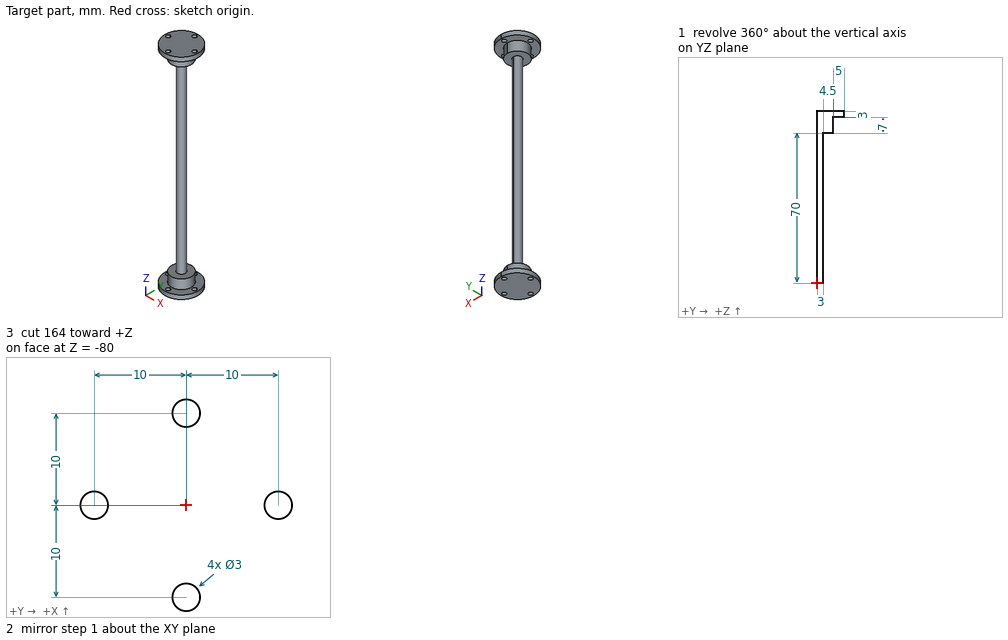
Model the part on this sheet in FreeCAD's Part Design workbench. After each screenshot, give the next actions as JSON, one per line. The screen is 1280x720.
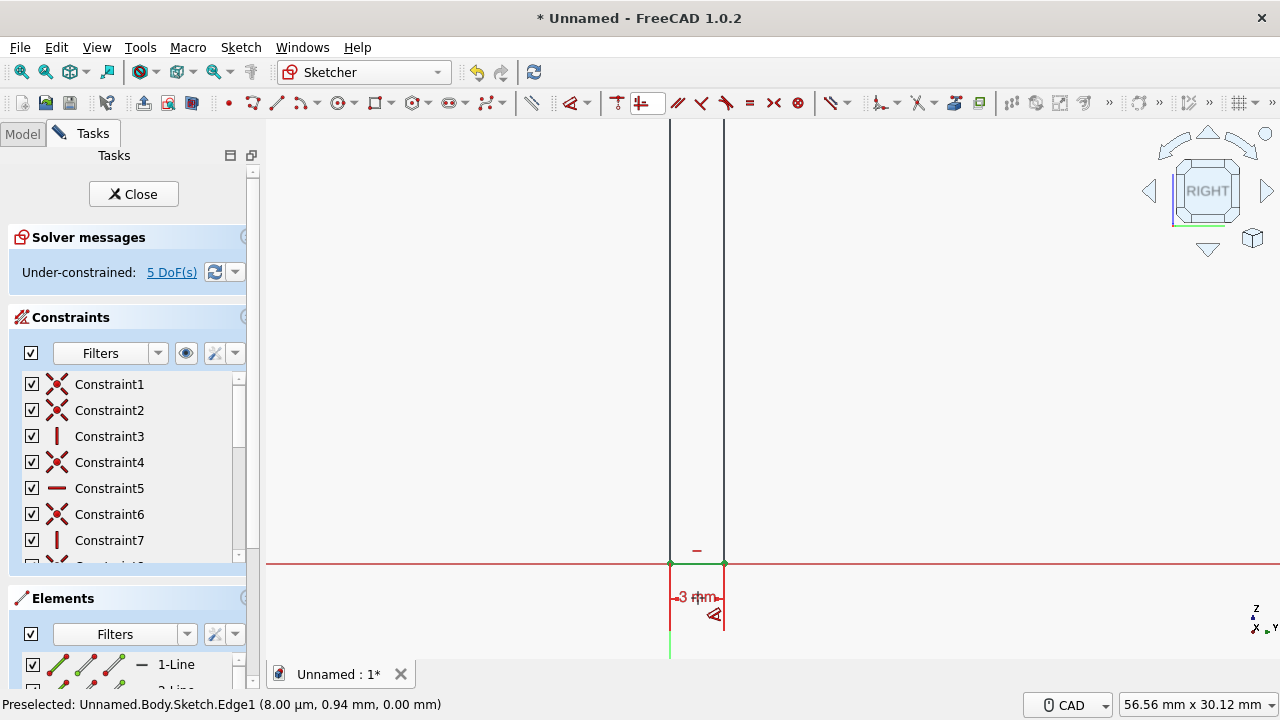
{"action": "scroll", "coordinate": [679, 567], "scroll_direction": "down", "scroll_amount": 7}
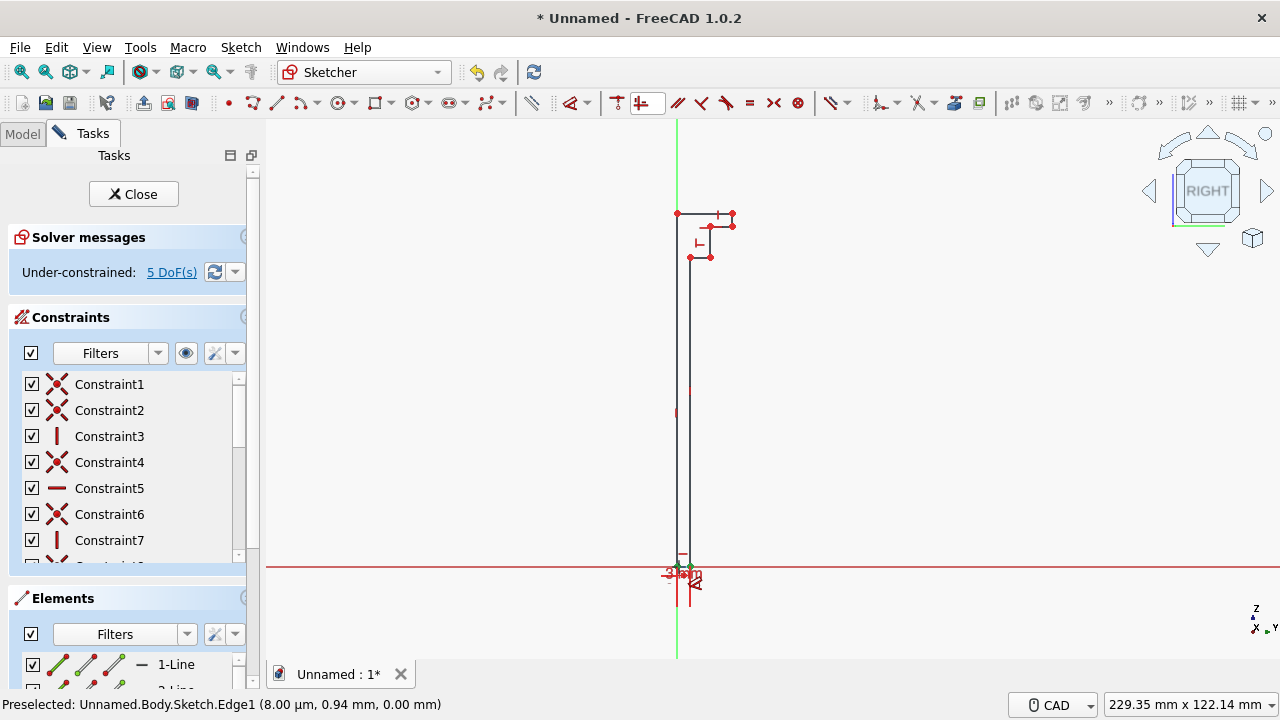
{"action": "scroll", "coordinate": [710, 249], "scroll_direction": "up", "scroll_amount": 2}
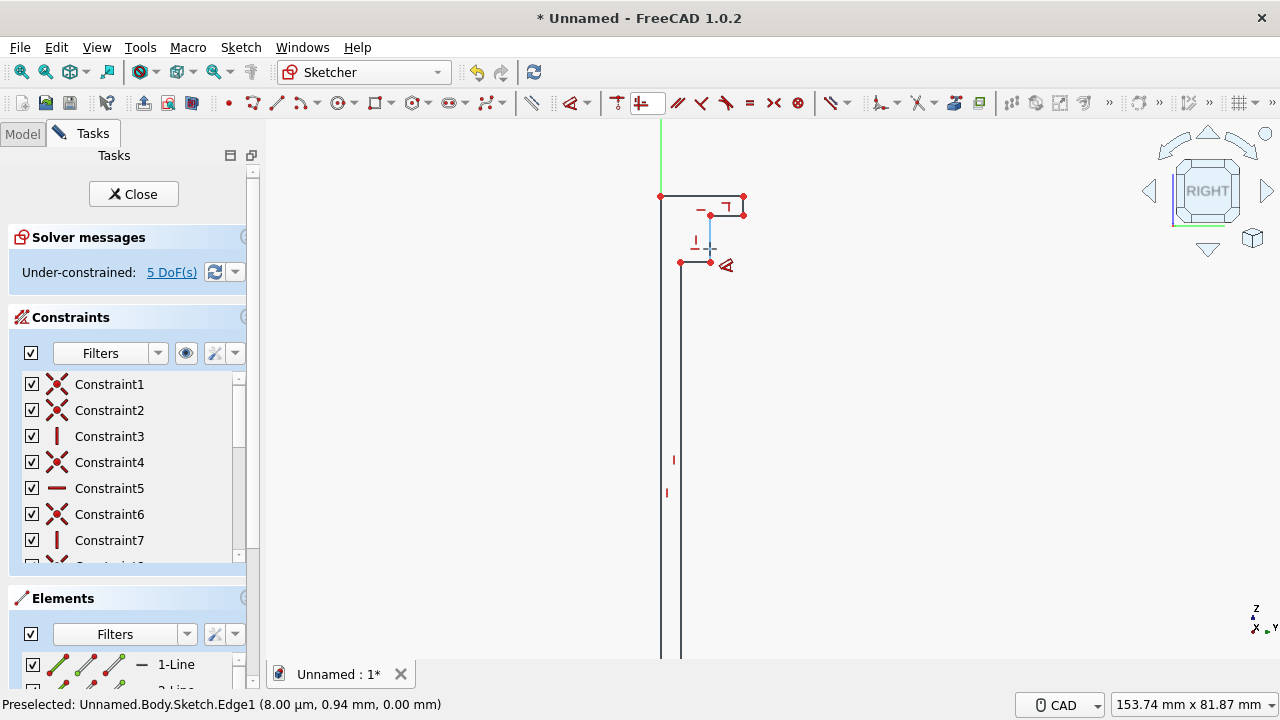
{"action": "left_click", "coordinate": [710, 248]}
{"action": "left_click", "coordinate": [744, 239]}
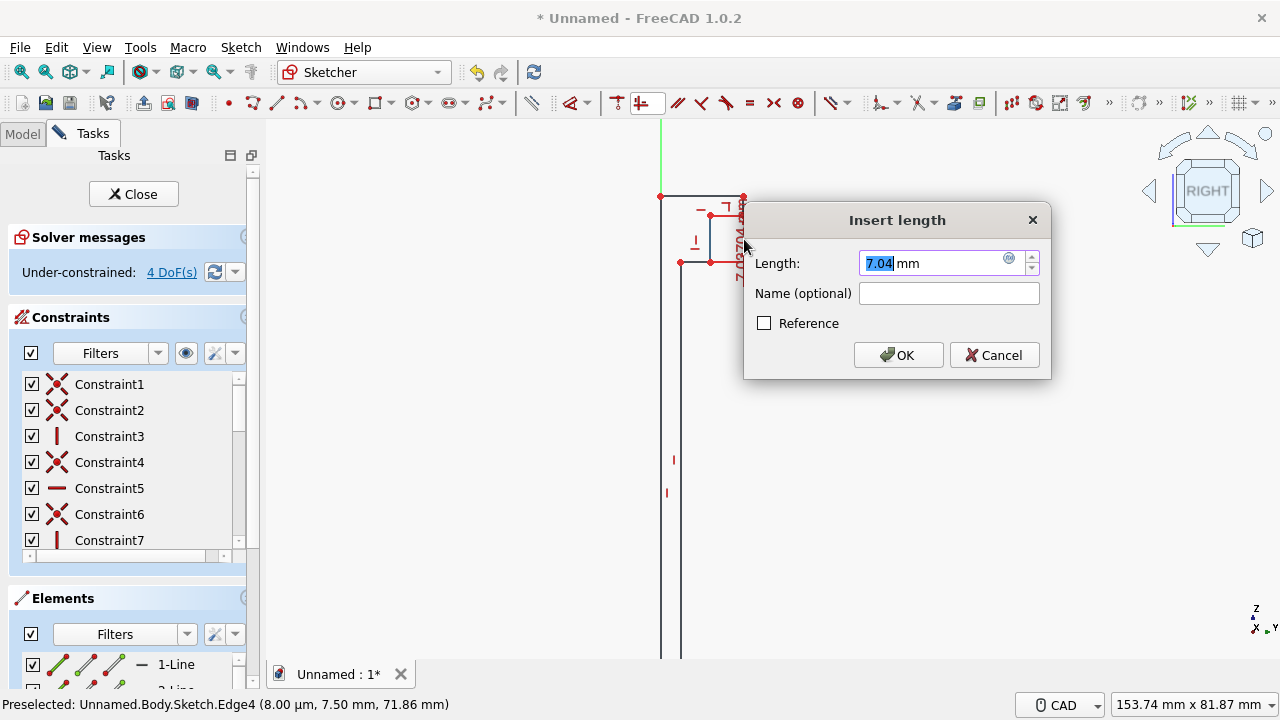
{"action": "type", "text": "7"}
{"action": "key", "text": "Return"}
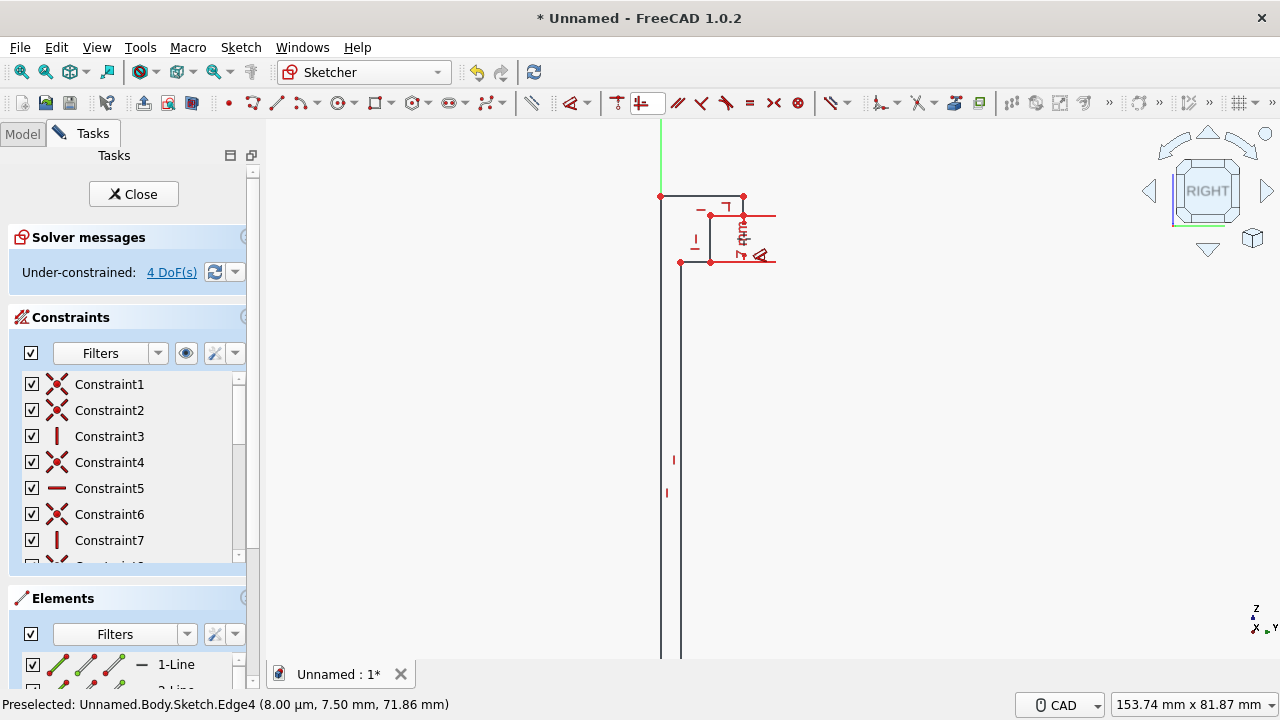
{"action": "scroll", "coordinate": [720, 216], "scroll_direction": "up", "scroll_amount": 2}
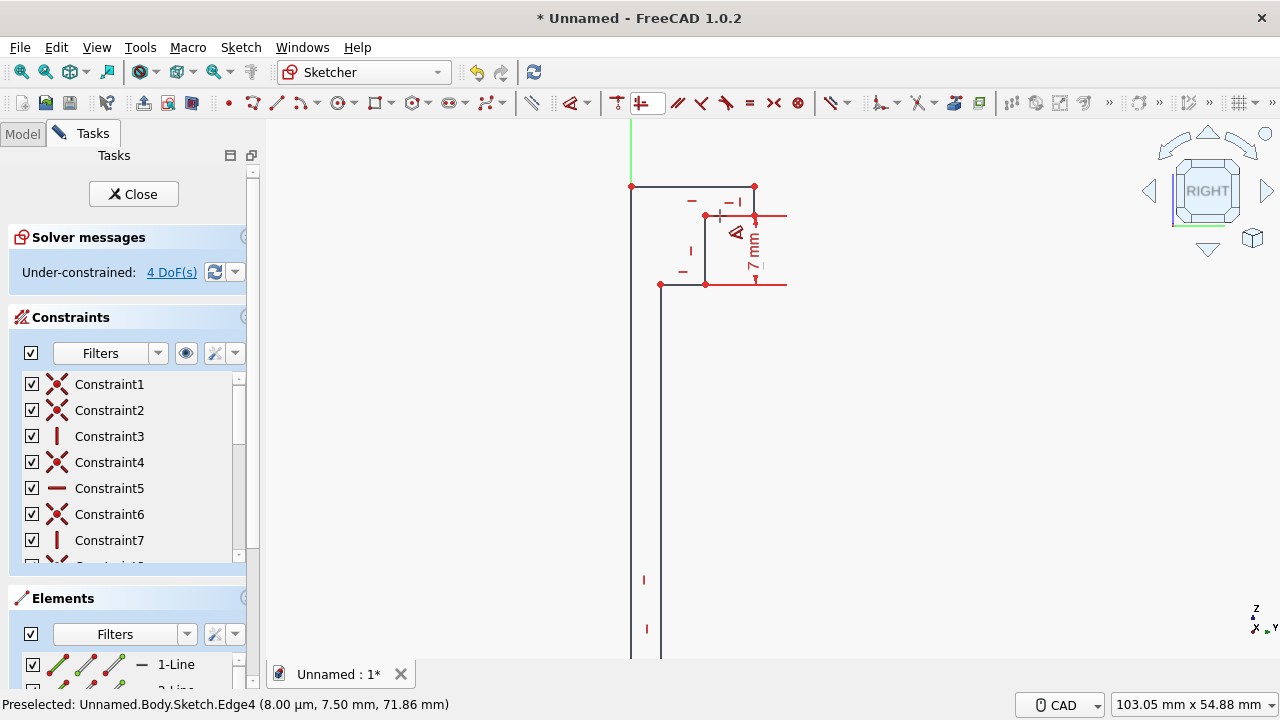
{"action": "left_click", "coordinate": [720, 216]}
{"action": "left_click", "coordinate": [730, 158]}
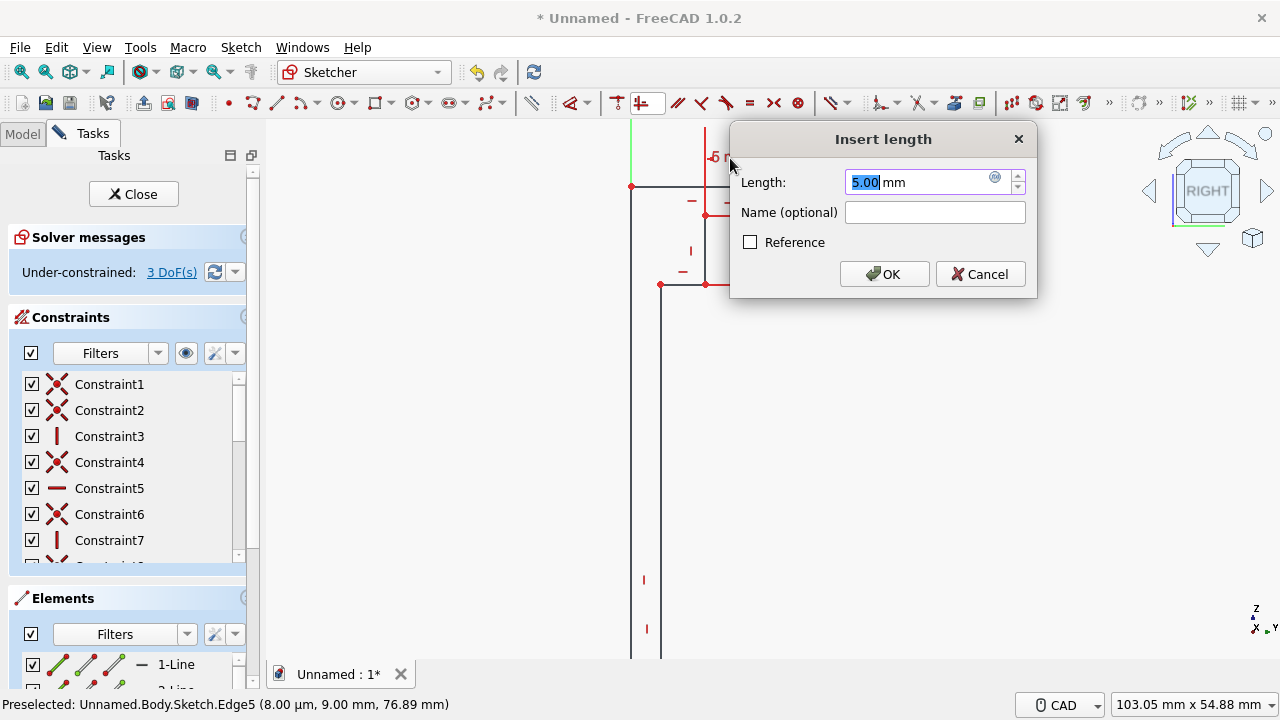
{"action": "type", "text": "5"}
{"action": "key", "text": "Return"}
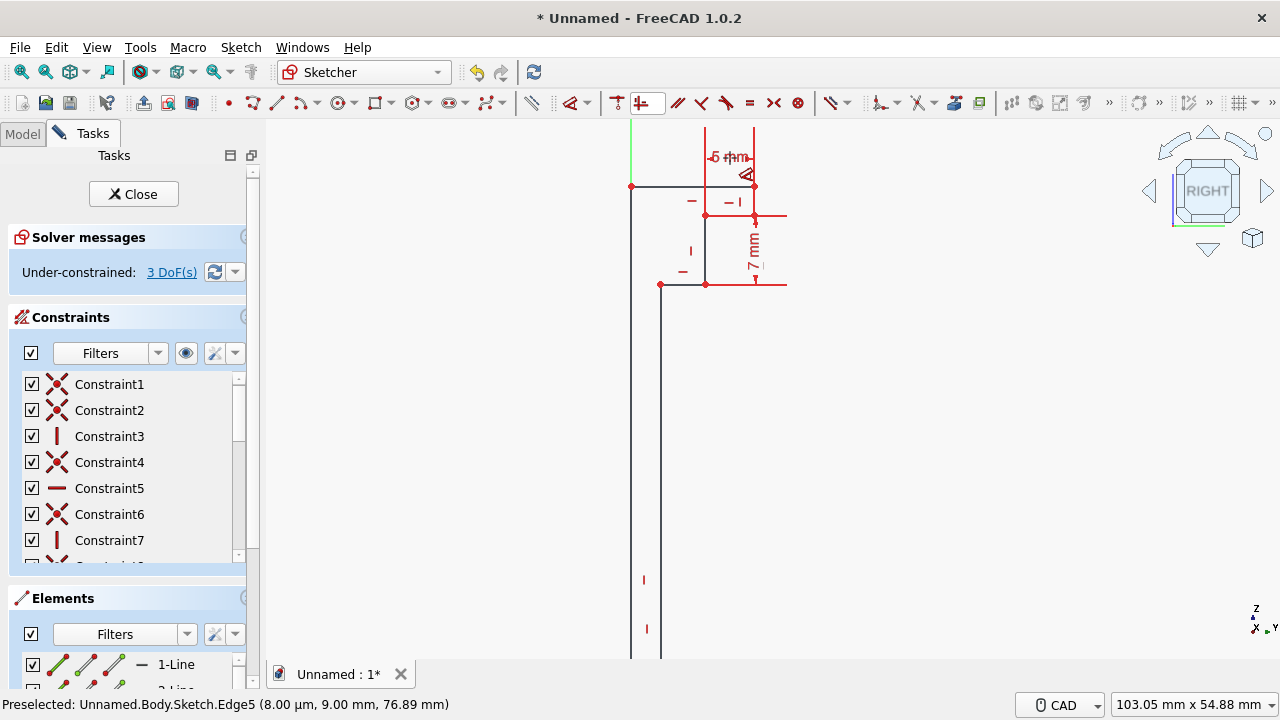
{"action": "scroll", "coordinate": [754, 204], "scroll_direction": "up", "scroll_amount": 2}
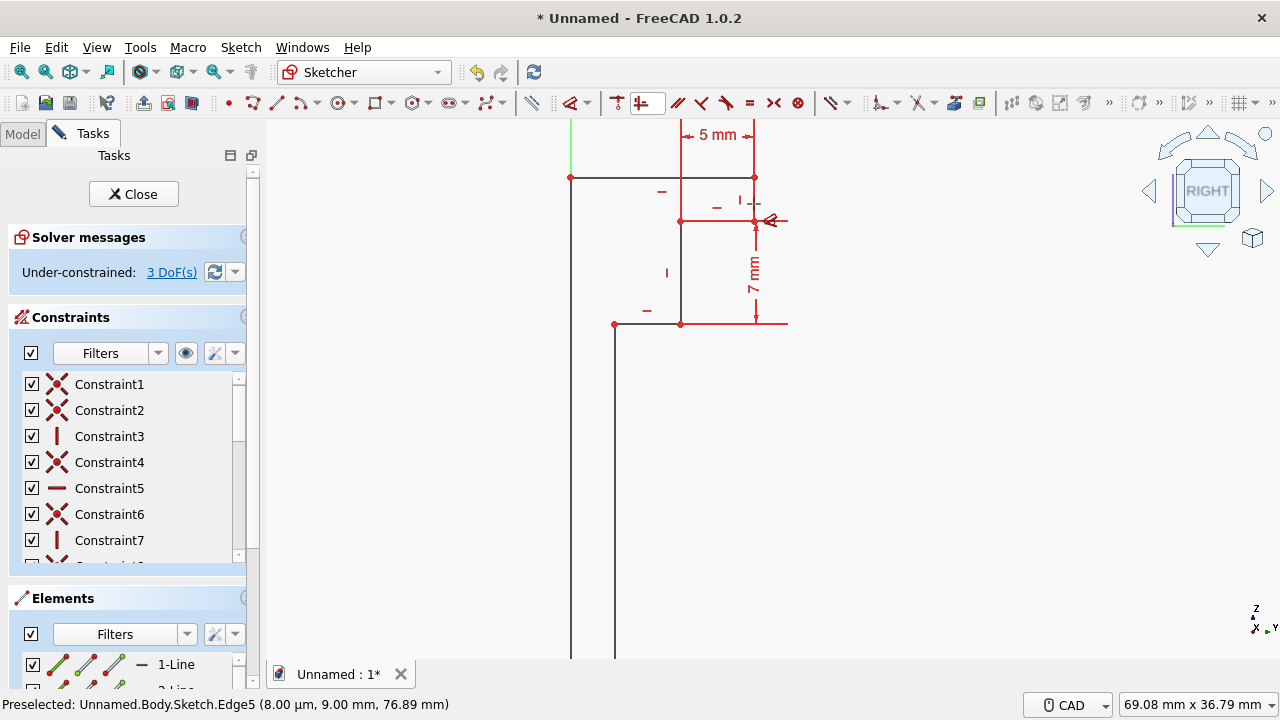
{"action": "left_click", "coordinate": [754, 204]}
{"action": "left_click", "coordinate": [788, 200]}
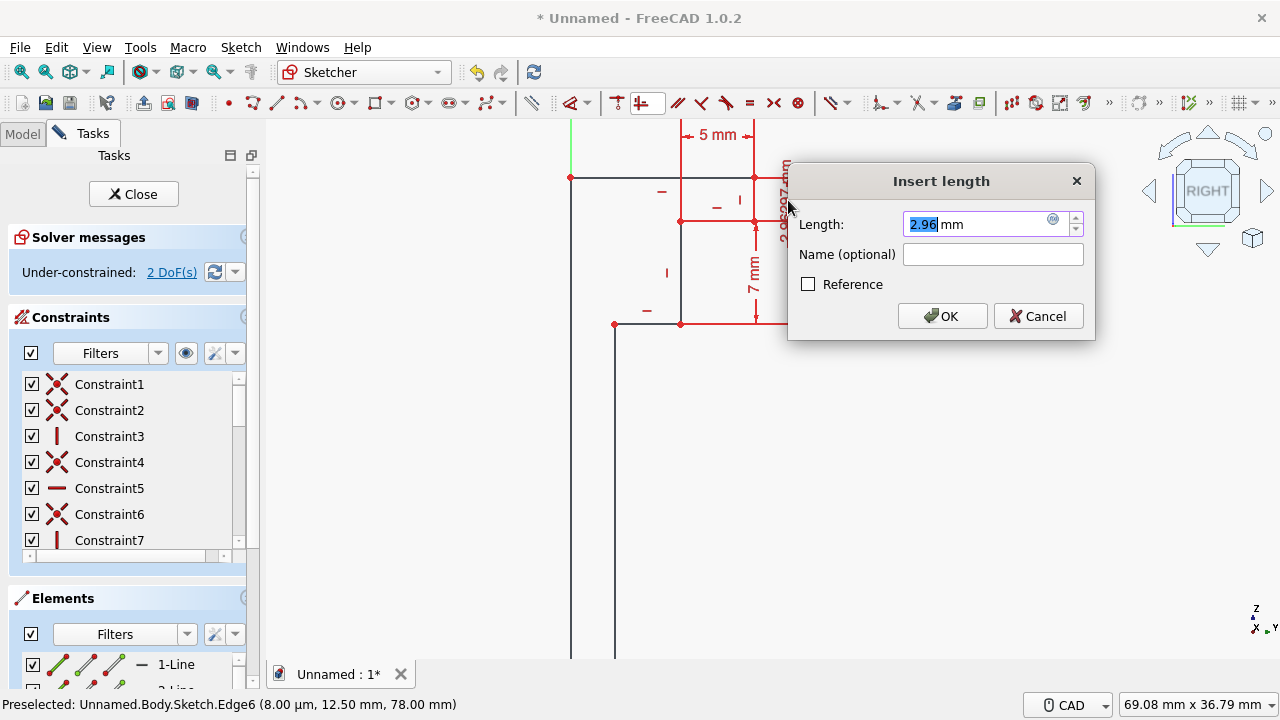
{"action": "type", "text": "3"}
{"action": "key", "text": "Return"}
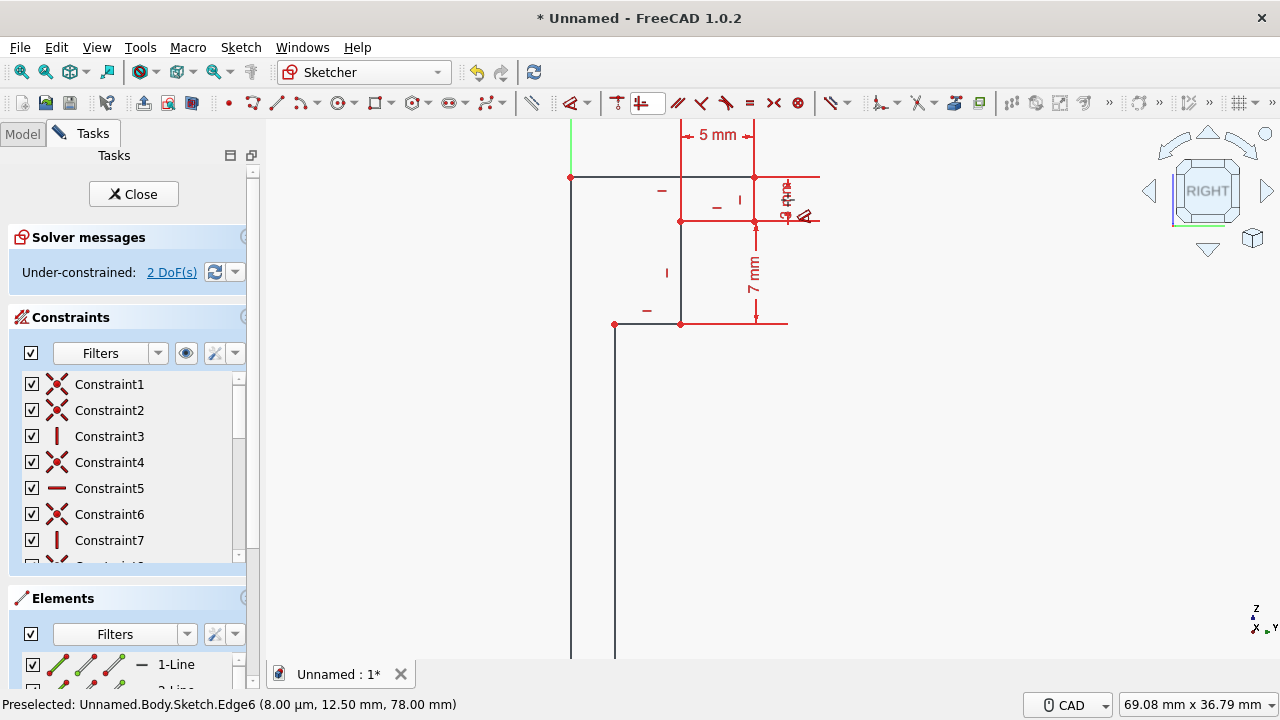
{"action": "scroll", "coordinate": [723, 228], "scroll_direction": "down", "scroll_amount": 6}